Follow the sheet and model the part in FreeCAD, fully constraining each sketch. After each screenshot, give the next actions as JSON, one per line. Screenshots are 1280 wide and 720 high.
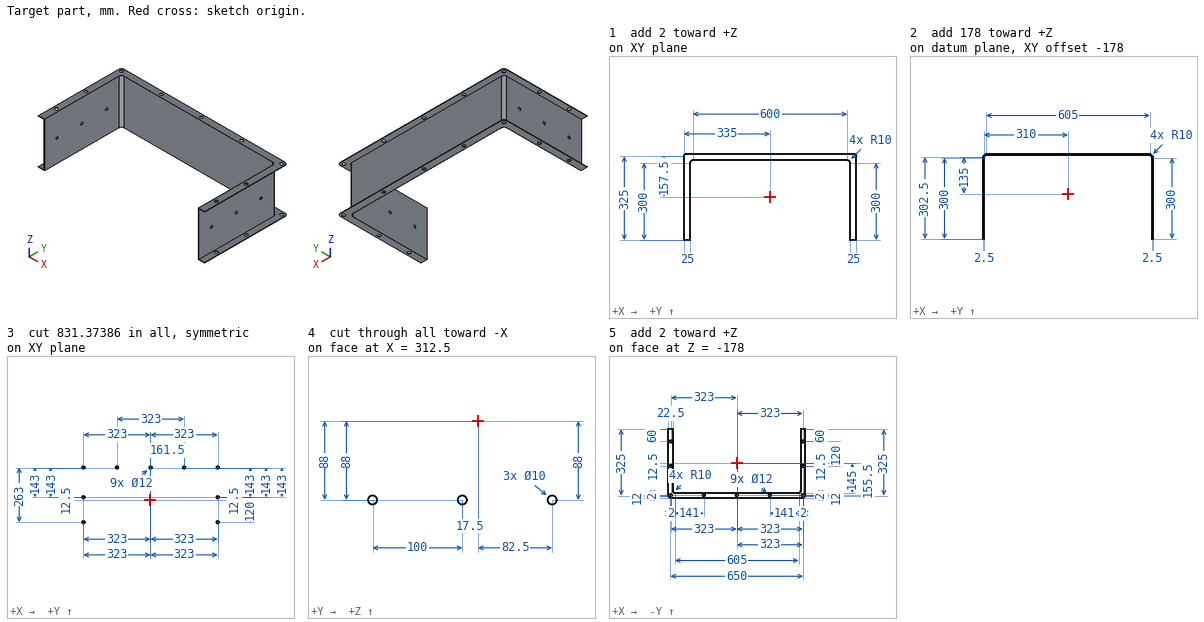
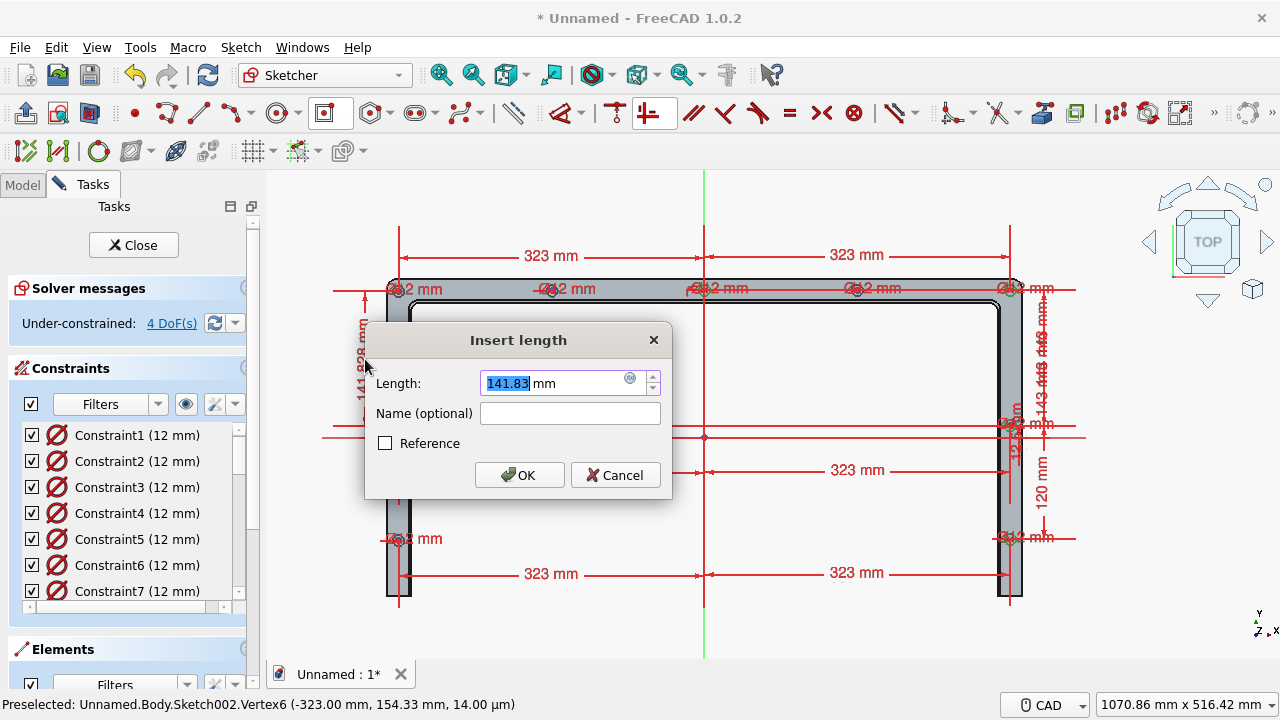
{"action": "type", "text": "143"}
{"action": "key", "text": "Return"}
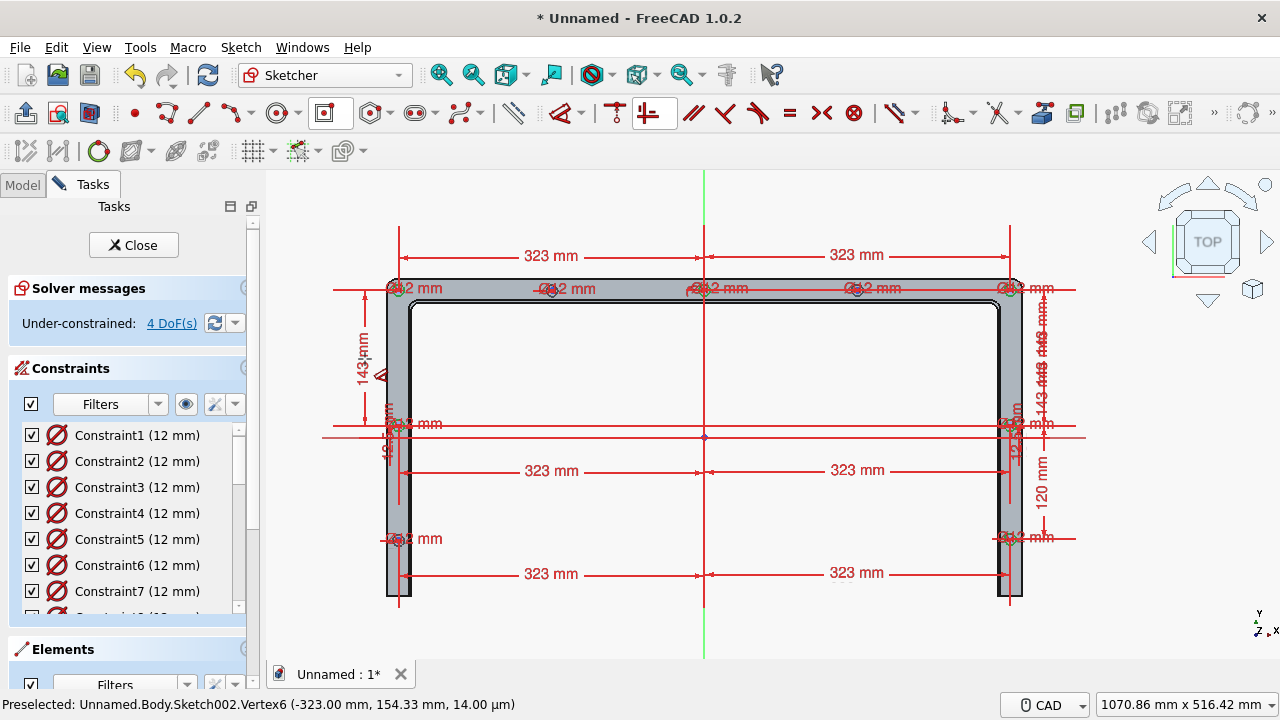
{"action": "left_click", "coordinate": [399, 290]}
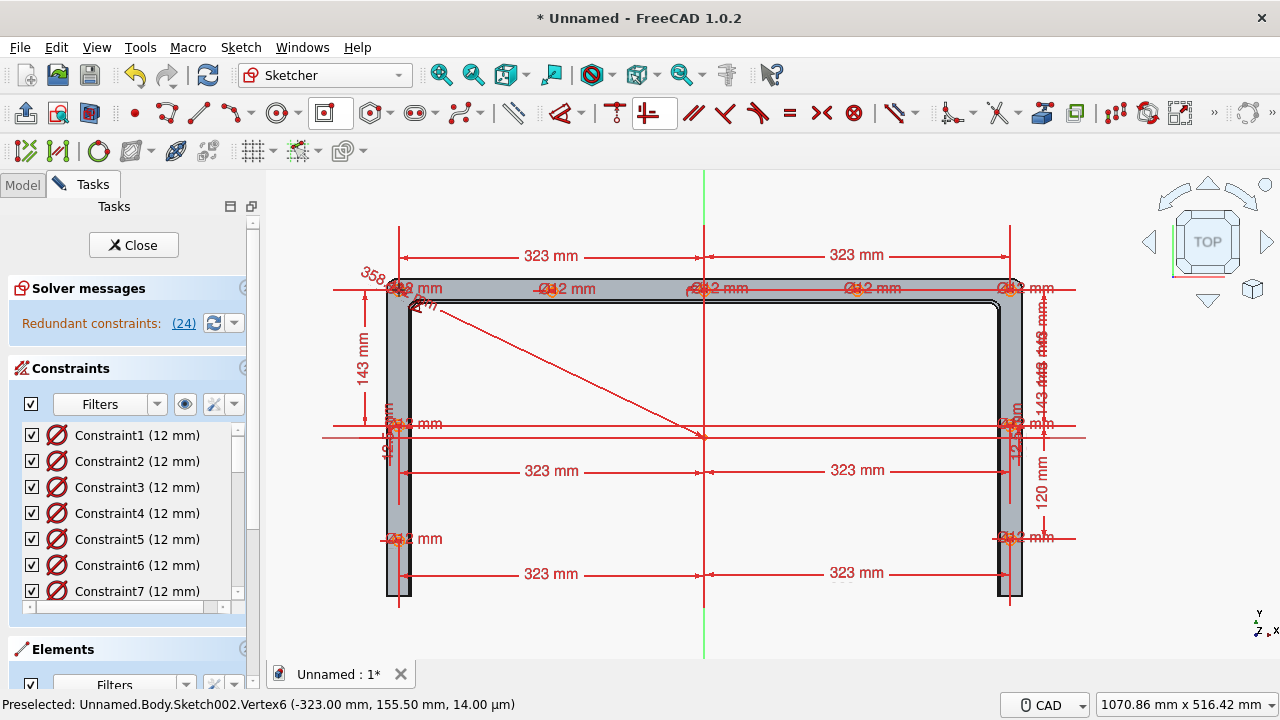
{"action": "left_click", "coordinate": [399, 541]}
{"action": "left_click", "coordinate": [365, 473]}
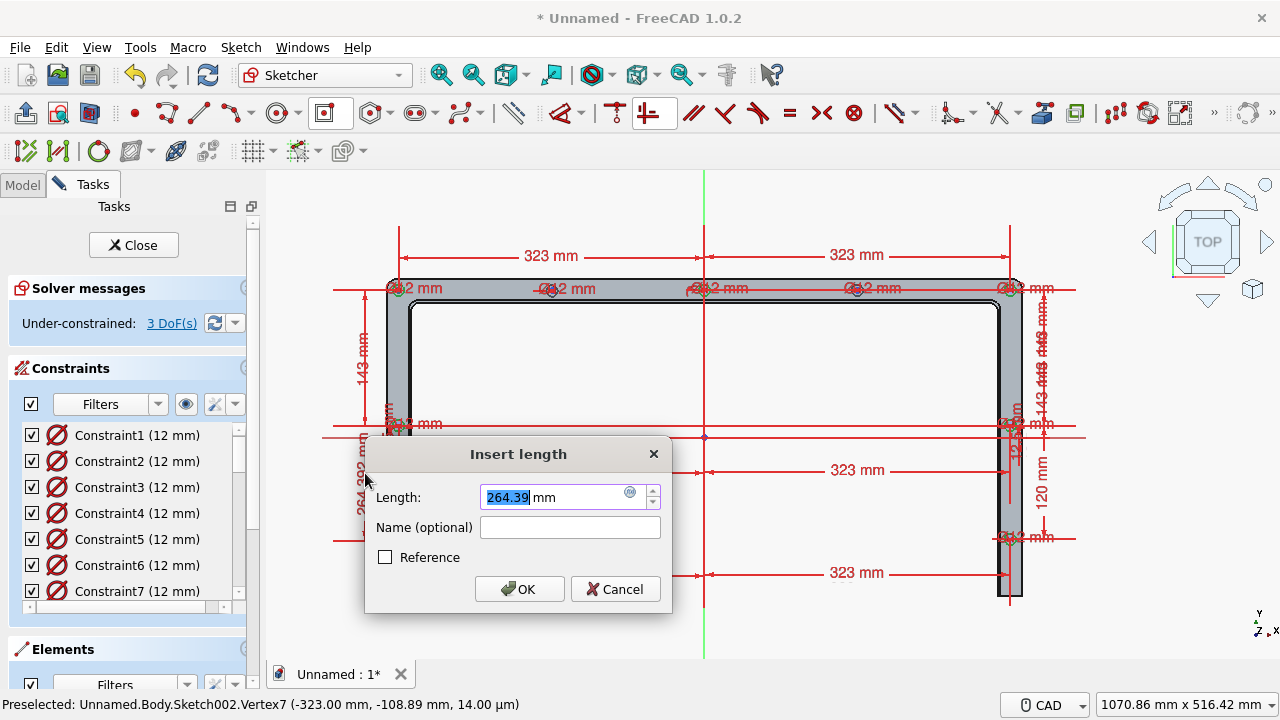
{"action": "type", "text": "263"}
{"action": "key", "text": "Return"}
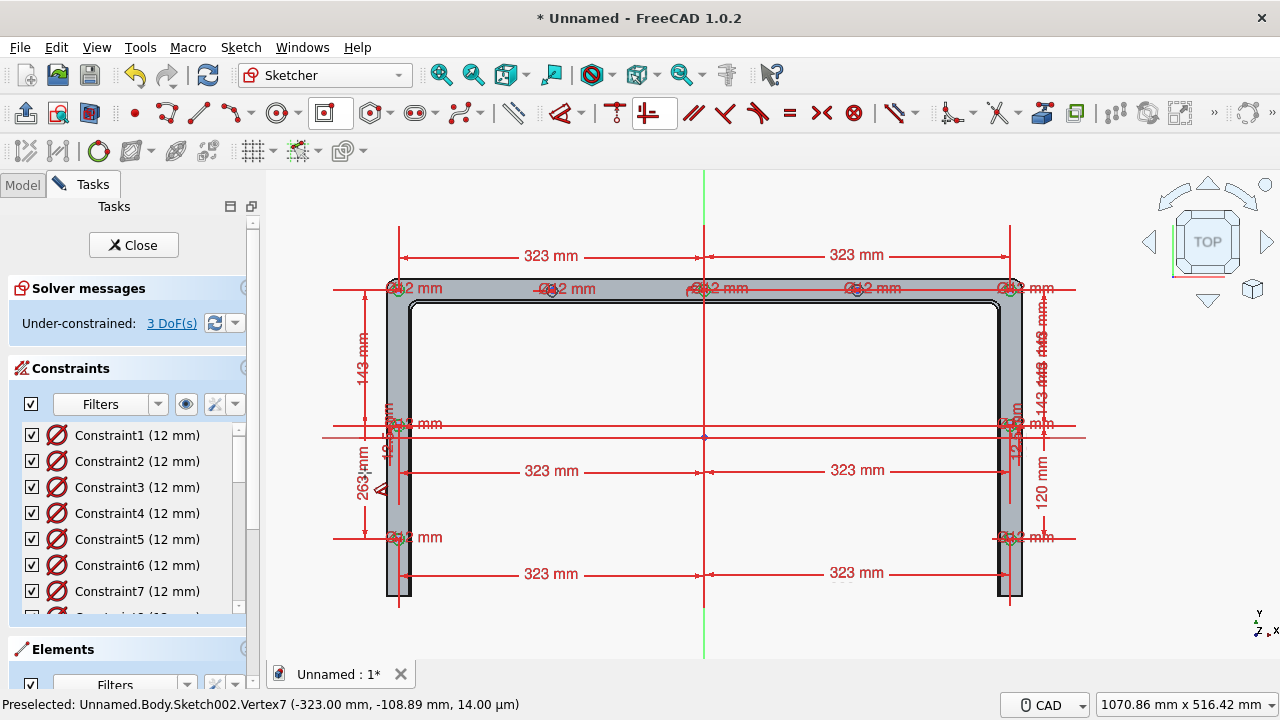
{"action": "left_click", "coordinate": [857, 290]}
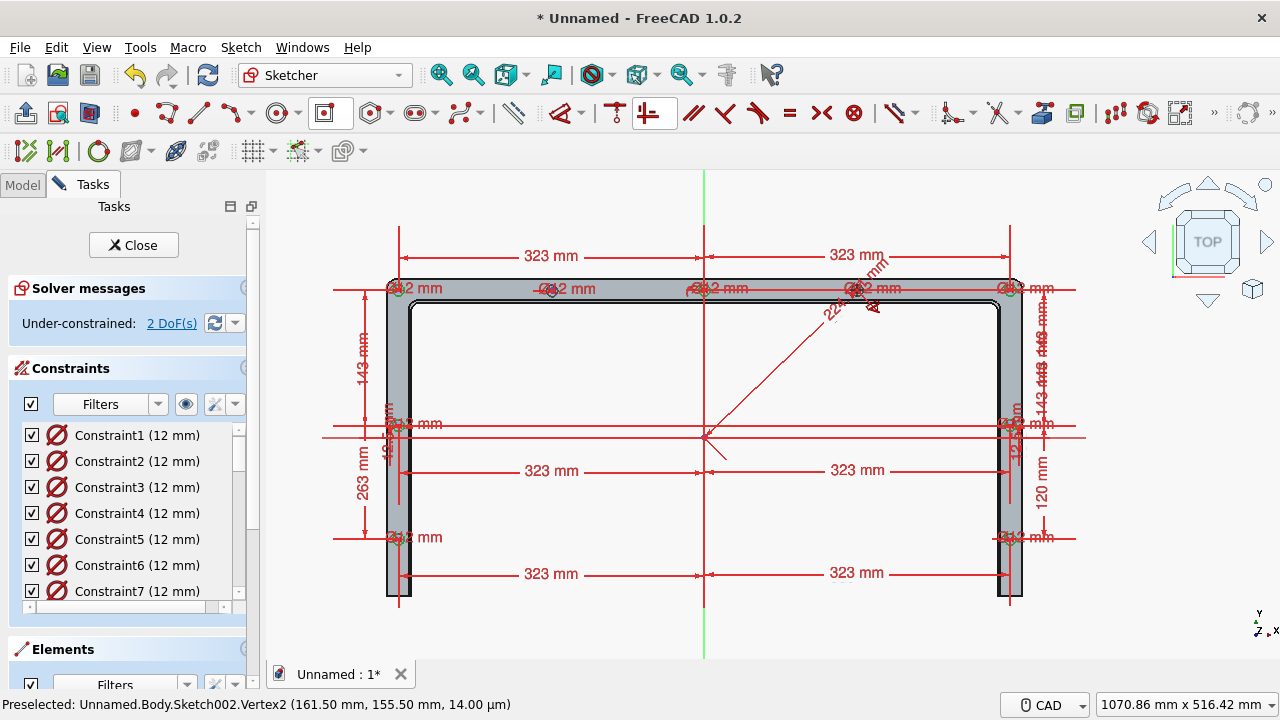
{"action": "left_click", "coordinate": [552, 291]}
{"action": "left_click", "coordinate": [634, 256]}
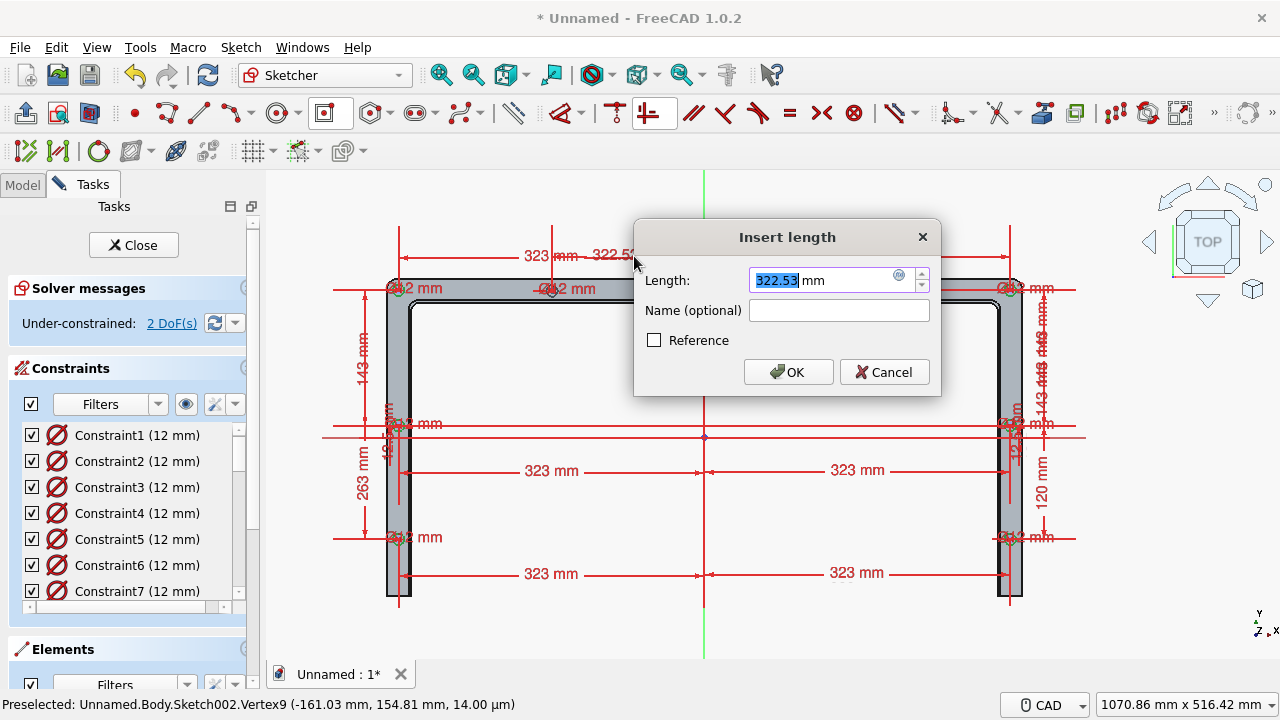
{"action": "type", "text": "323"}
{"action": "key", "text": "Return"}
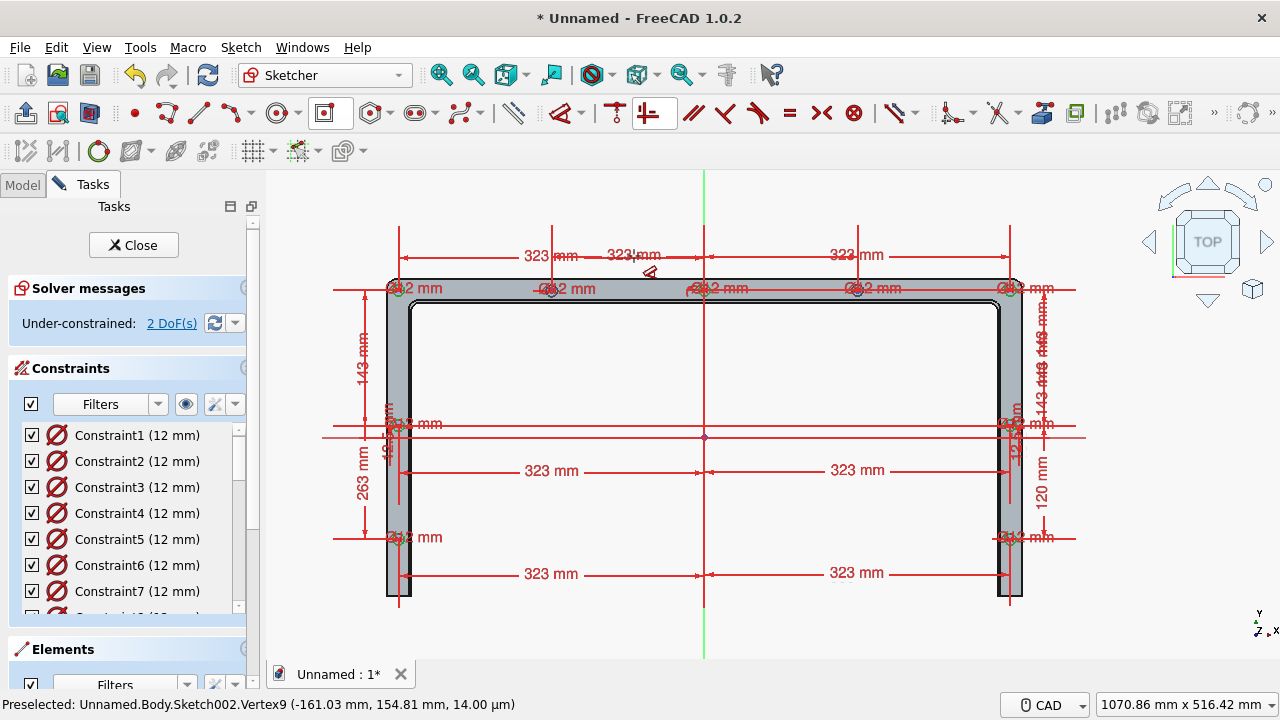
{"action": "left_click", "coordinate": [399, 426]}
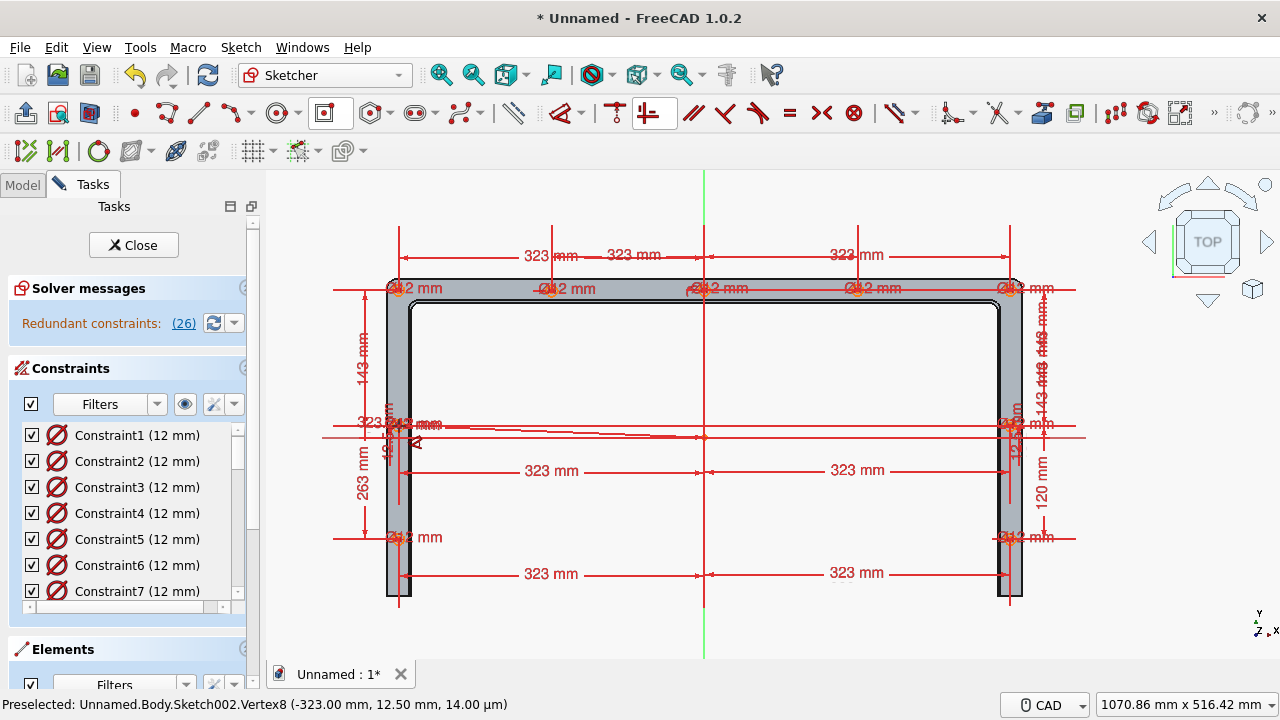
{"action": "left_click", "coordinate": [552, 291]}
{"action": "left_click", "coordinate": [365, 327]}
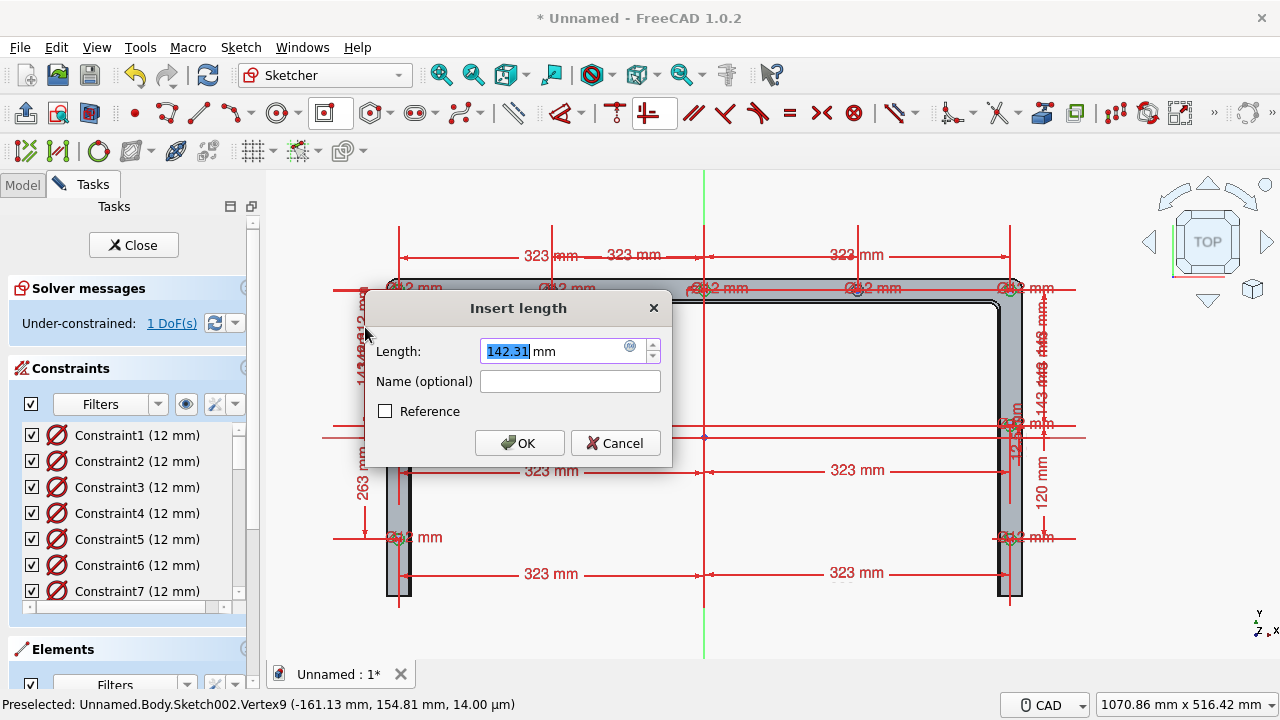
{"action": "type", "text": "143"}
{"action": "key", "text": "Return"}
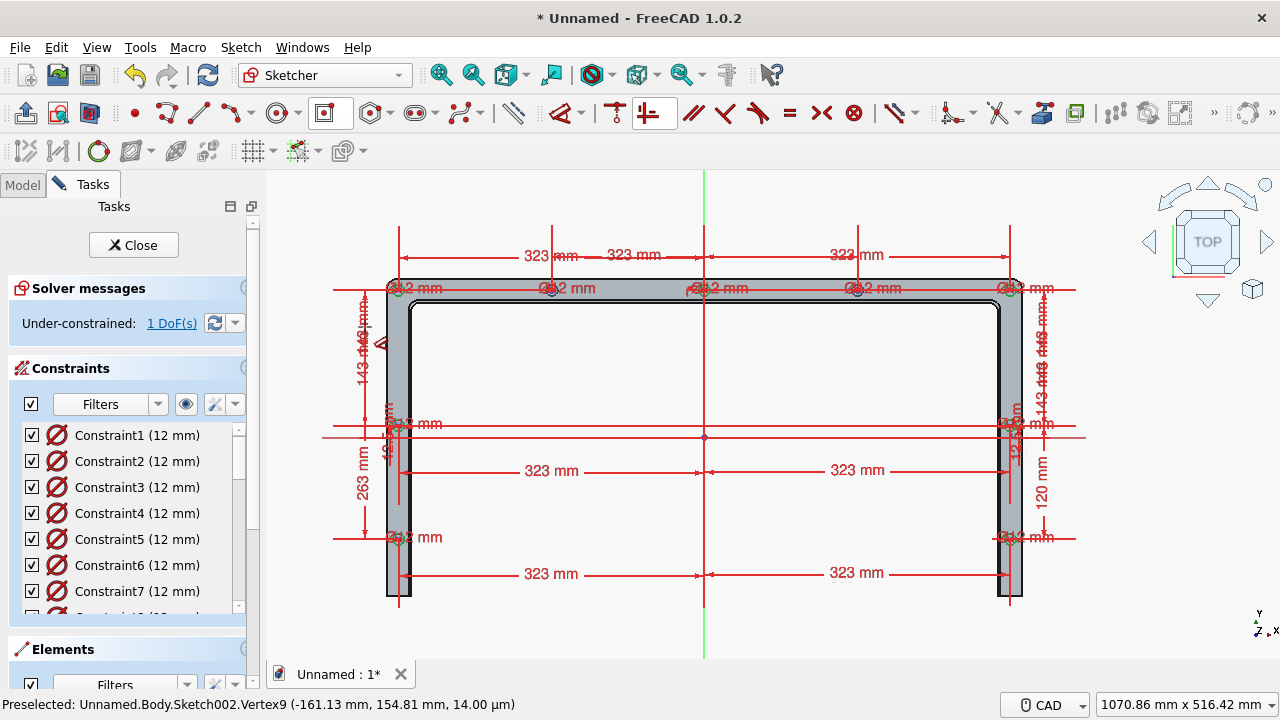
{"action": "left_click", "coordinate": [858, 290]}
{"action": "left_click", "coordinate": [781, 256]}